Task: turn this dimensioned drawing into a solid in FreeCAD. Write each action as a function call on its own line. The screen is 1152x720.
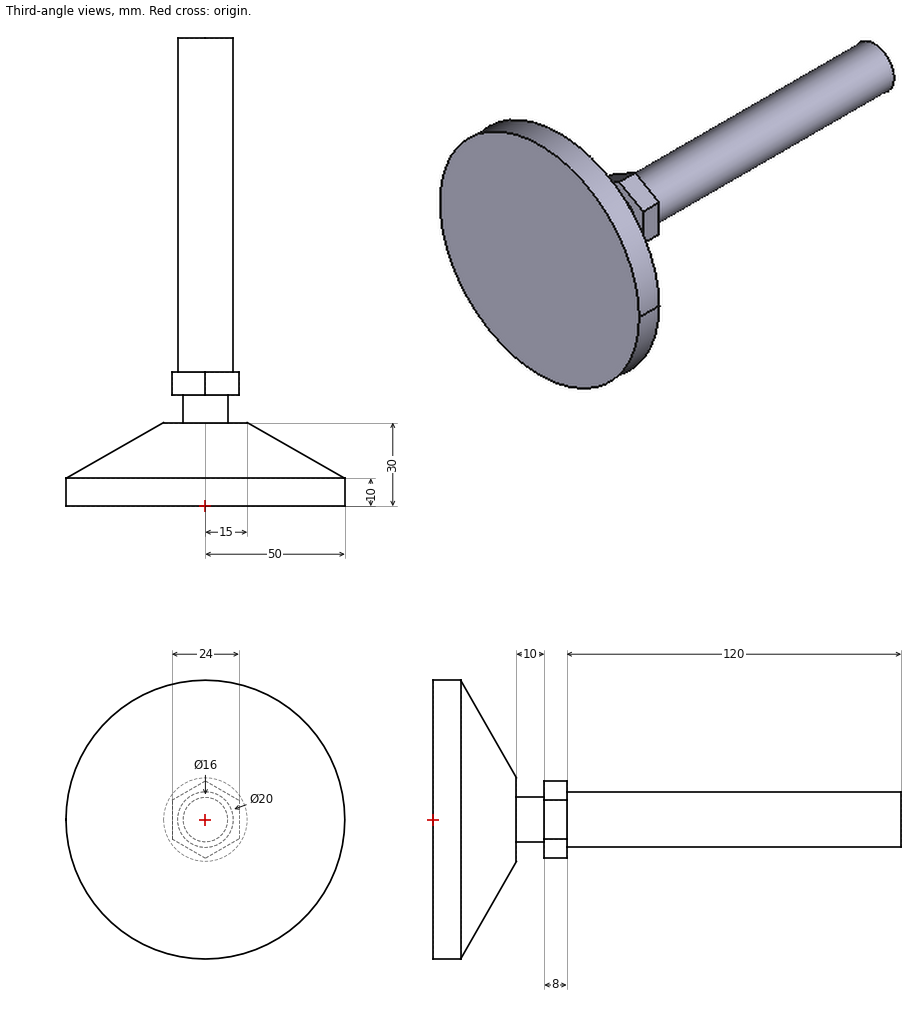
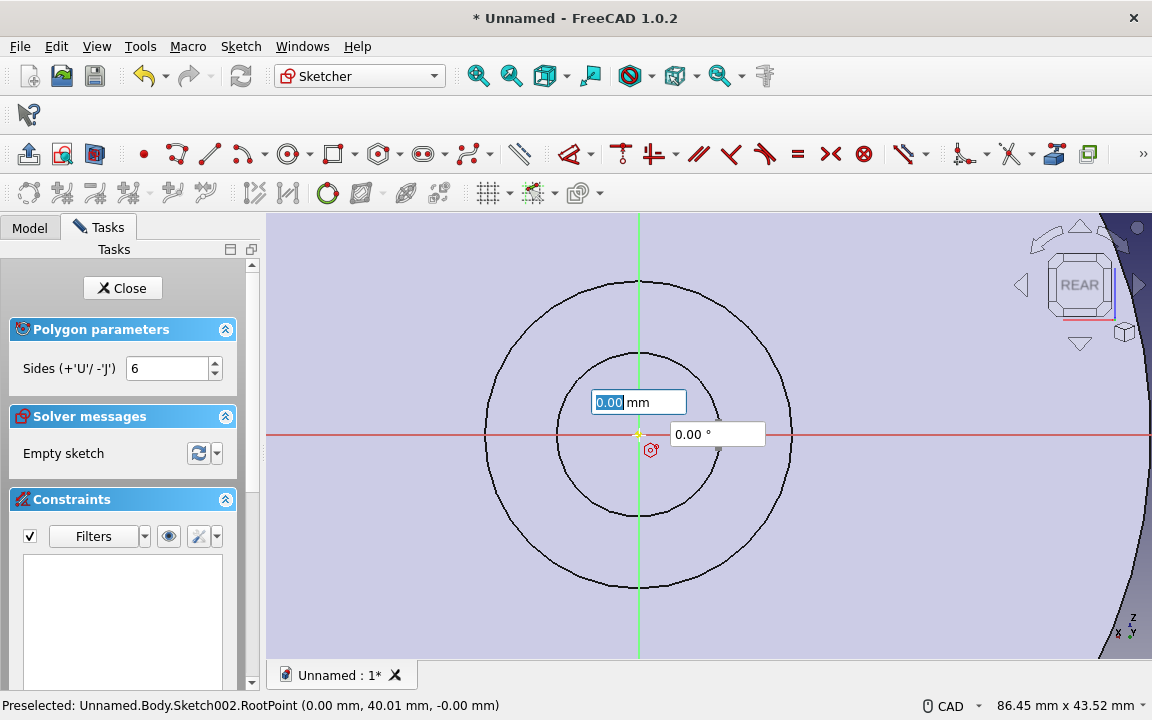
click(639, 577)
right_click(639, 577)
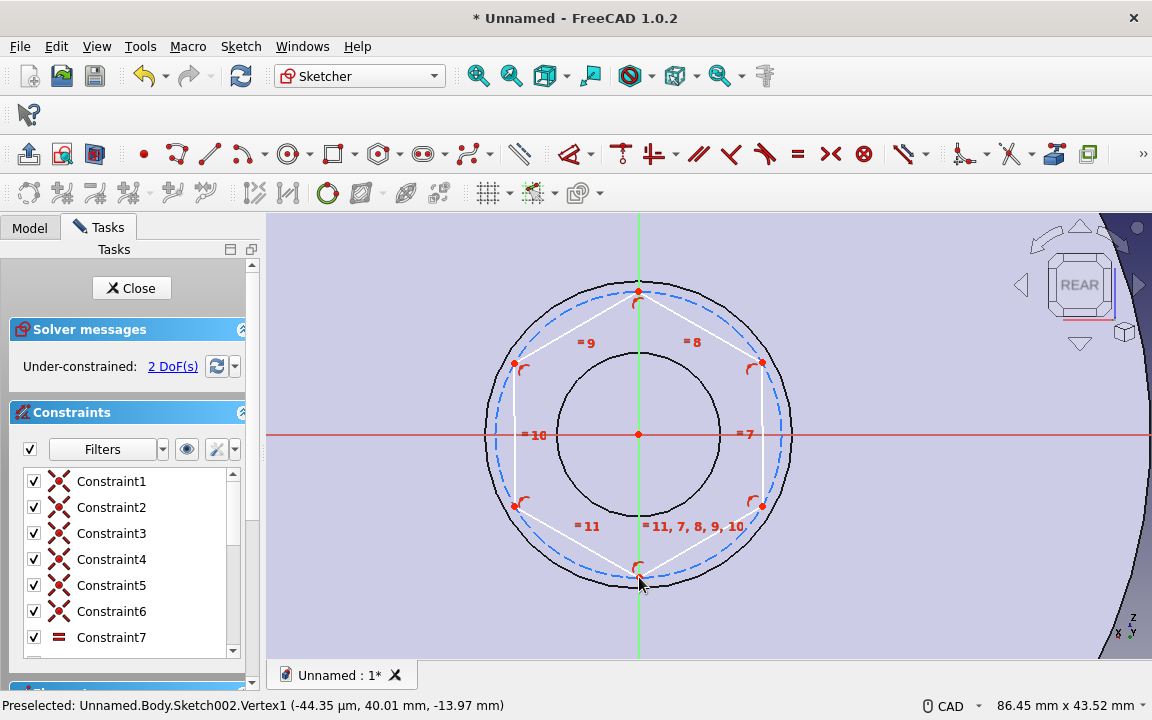
click(763, 463)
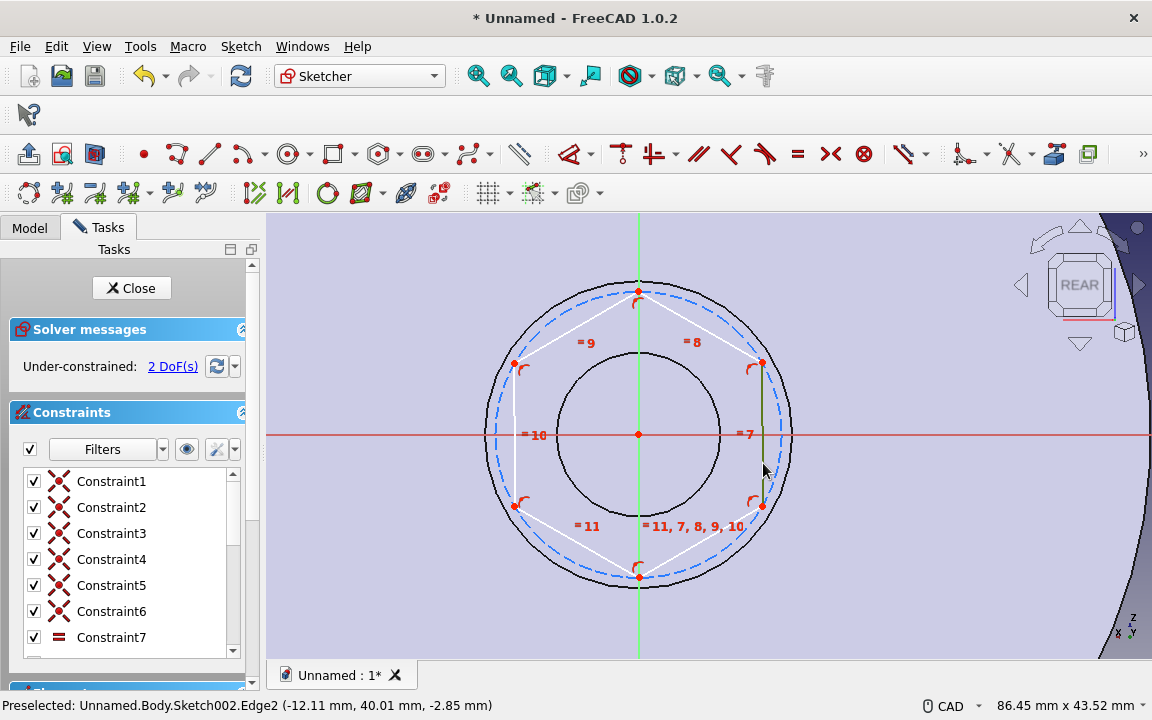
key(v)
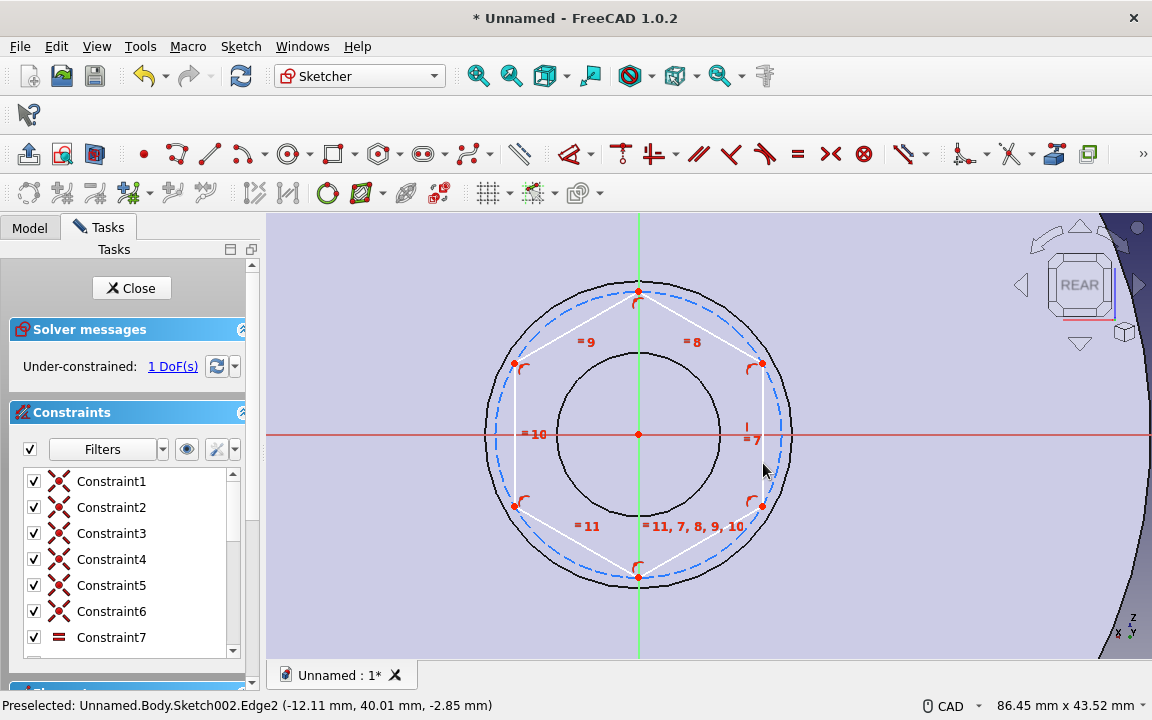
click(568, 154)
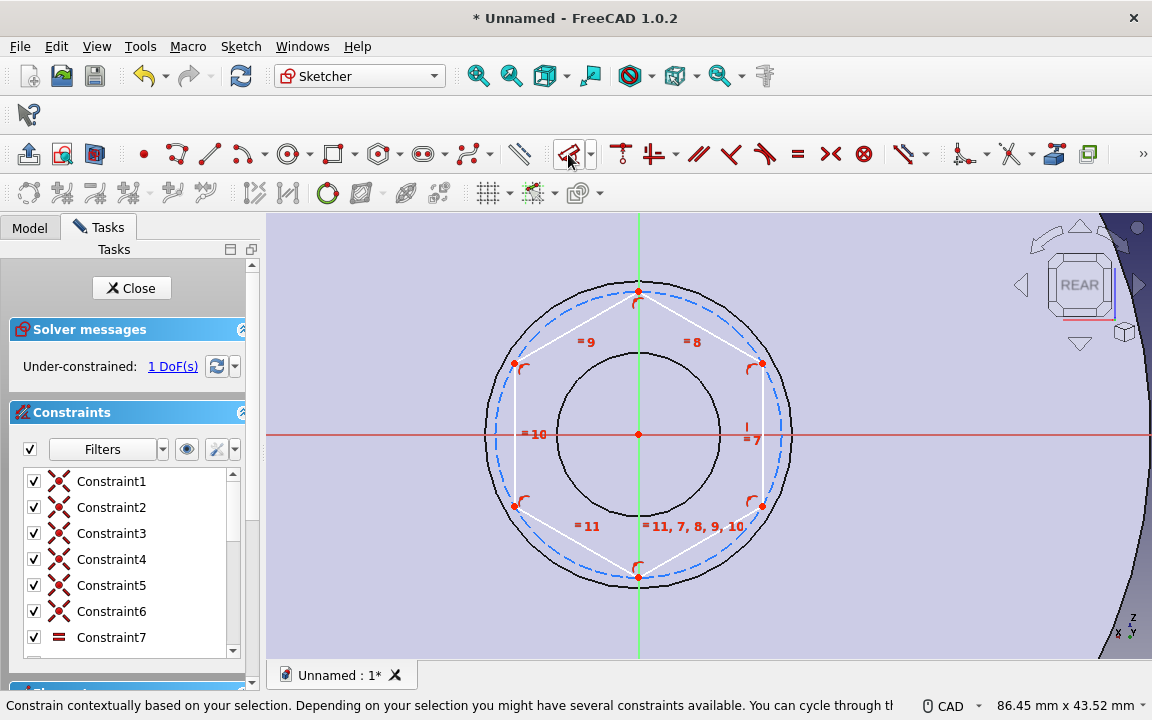
click(515, 363)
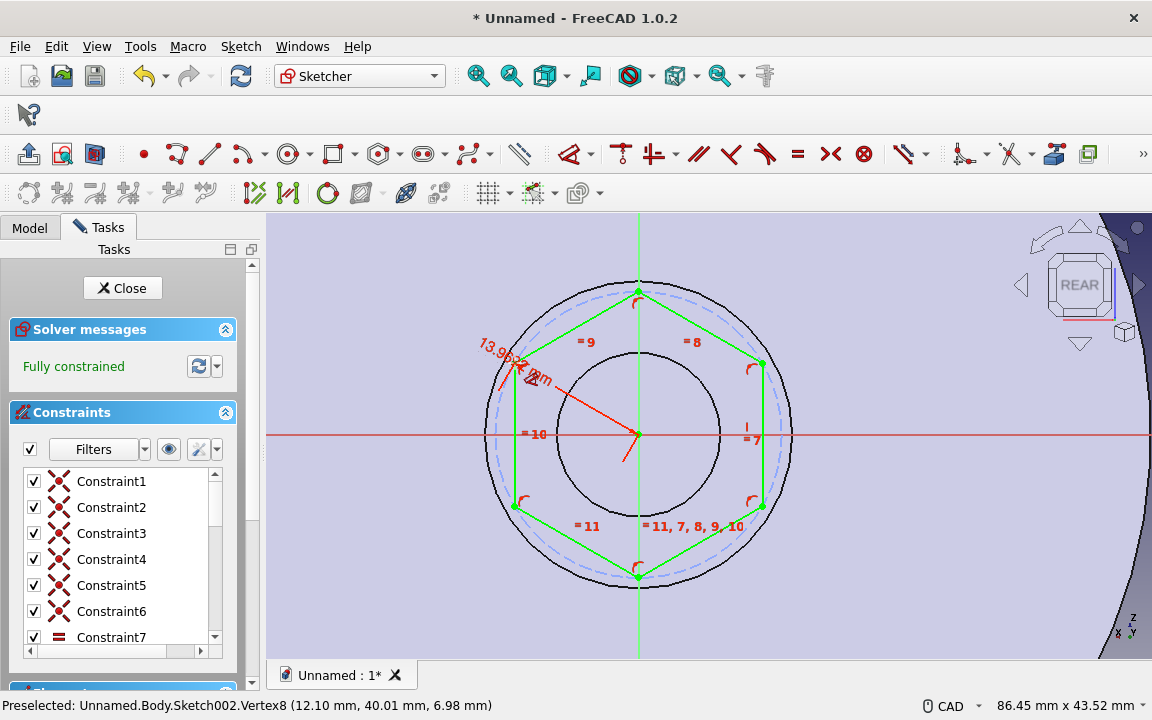
click(763, 506)
click(582, 588)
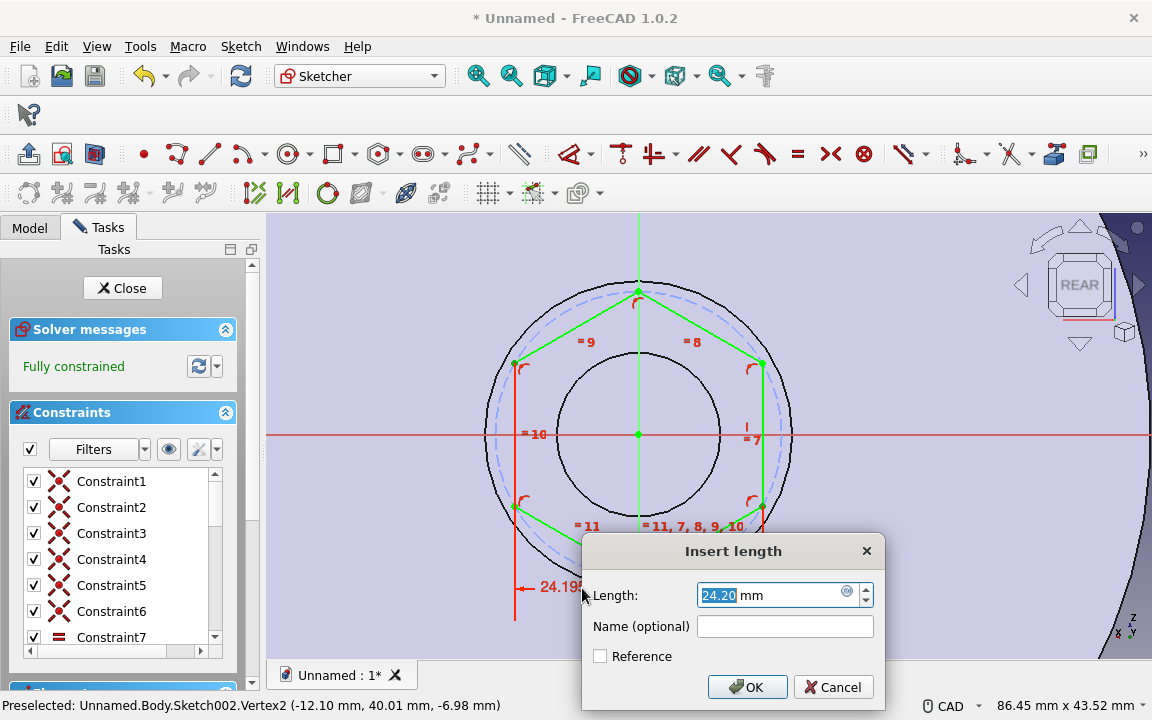
text(24)
key(Return)
key(Escape)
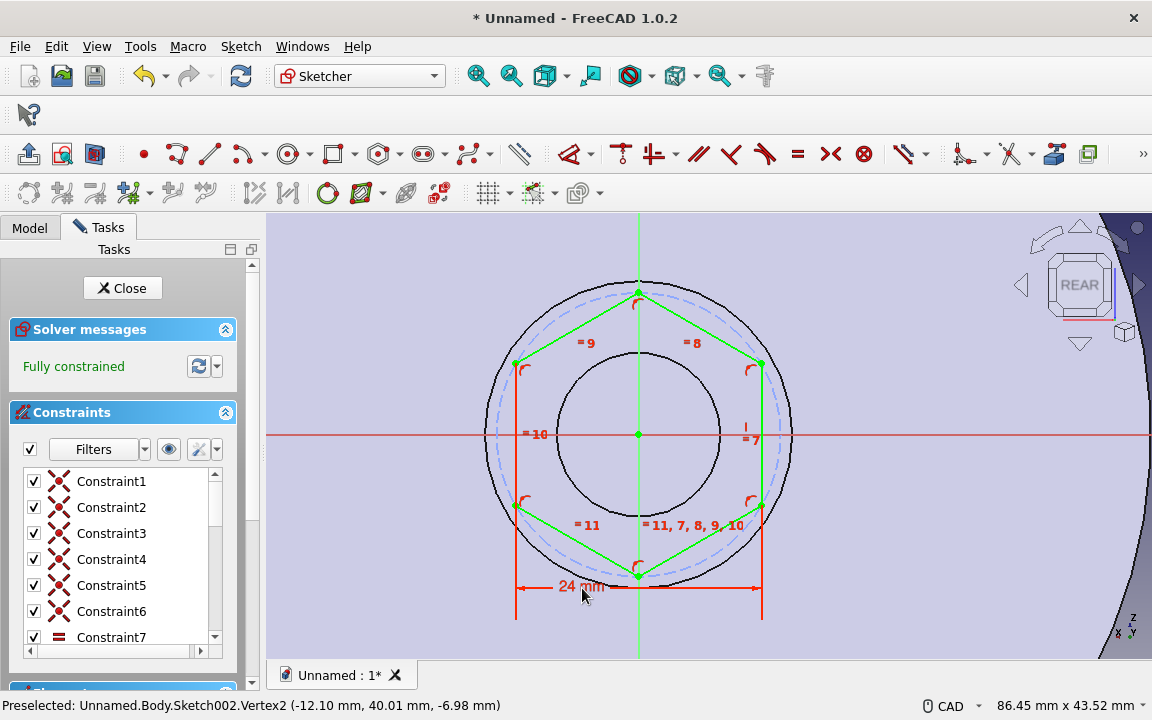
click(123, 288)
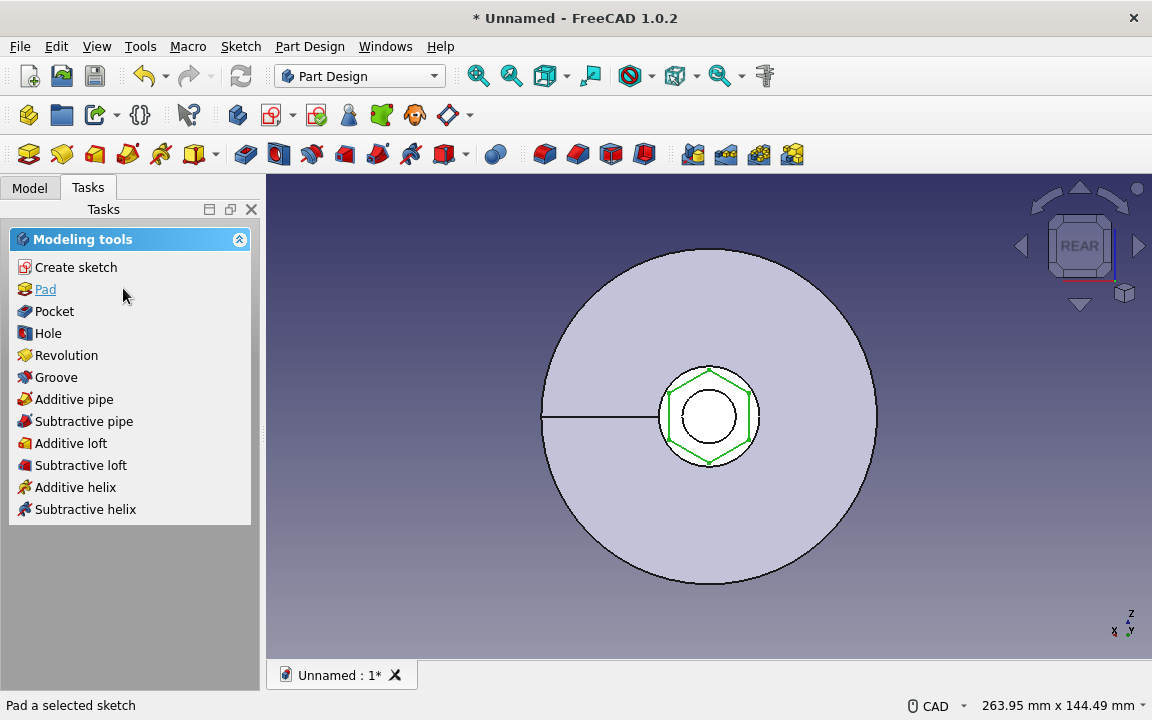
click(29, 154)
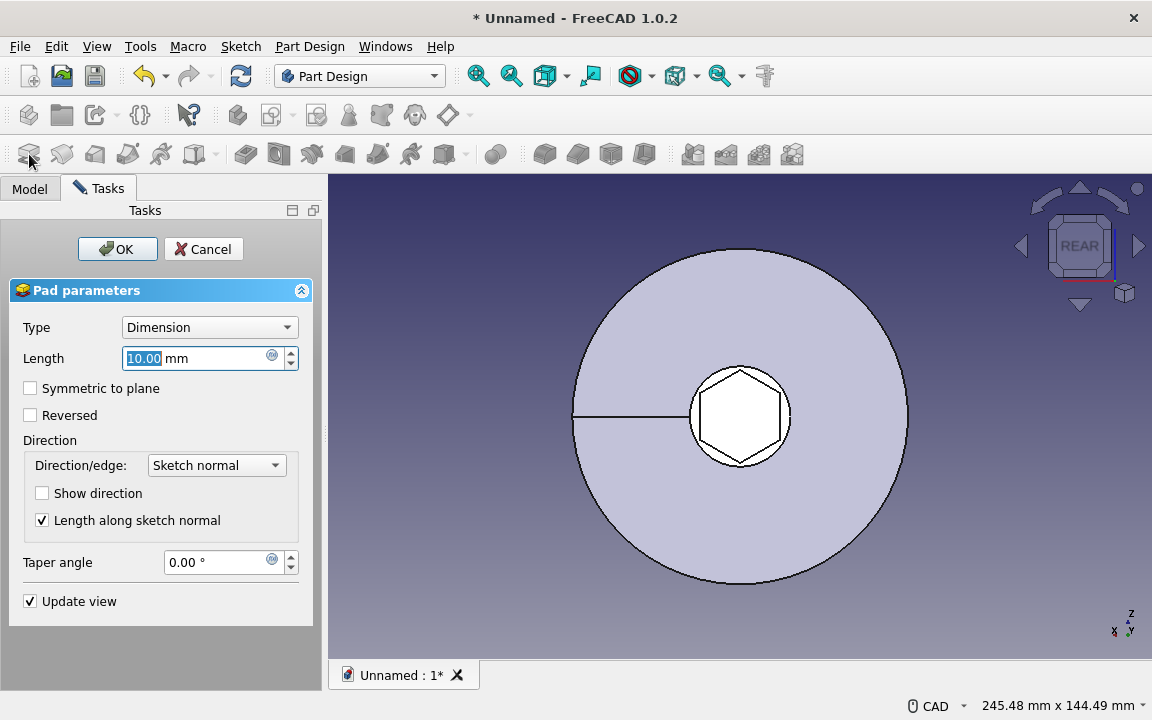
text(8)
key(Tab)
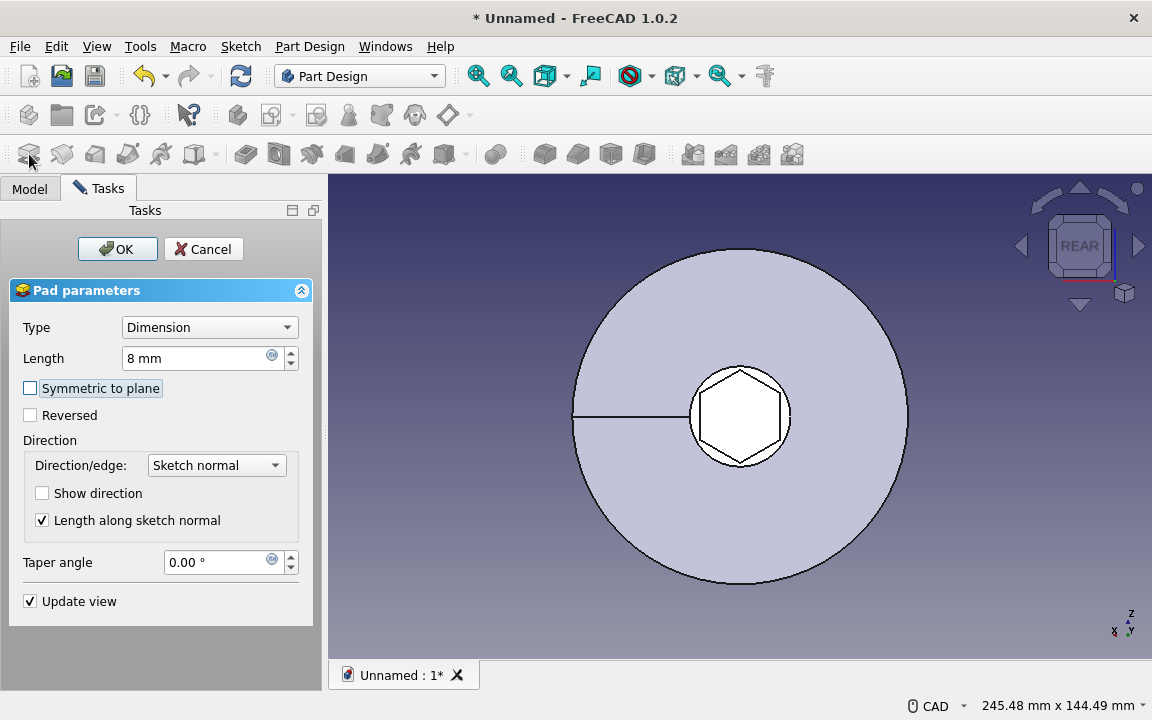
click(118, 249)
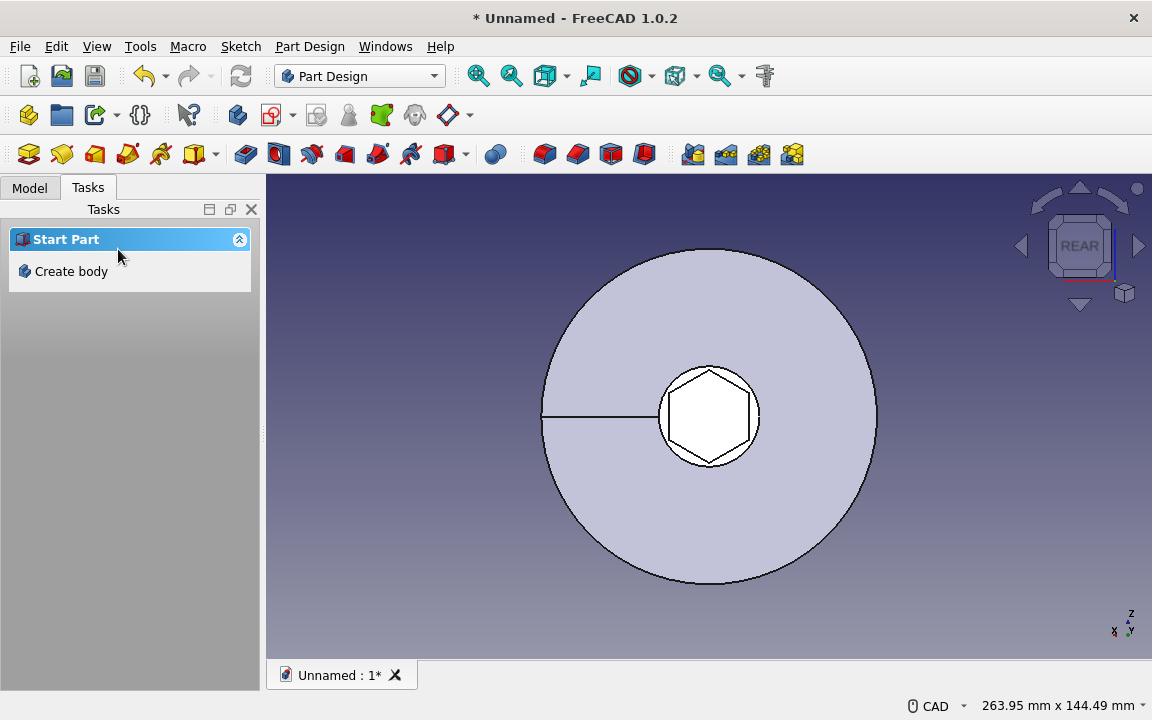
click(709, 415)